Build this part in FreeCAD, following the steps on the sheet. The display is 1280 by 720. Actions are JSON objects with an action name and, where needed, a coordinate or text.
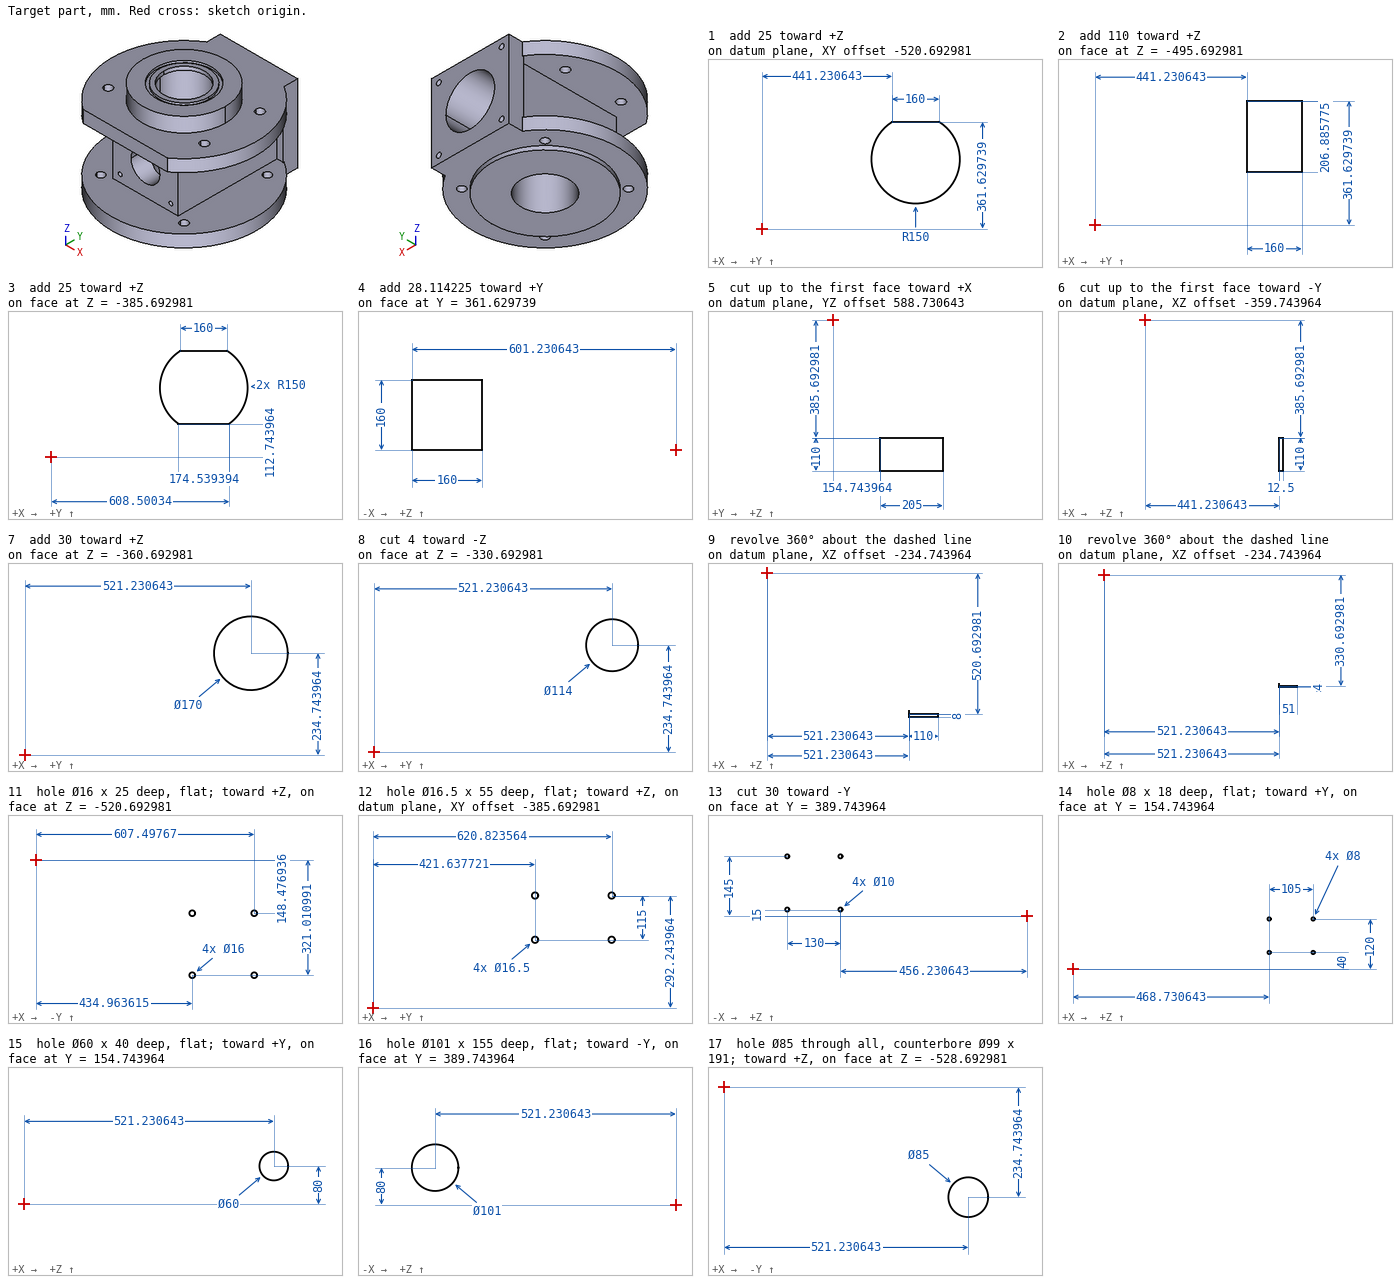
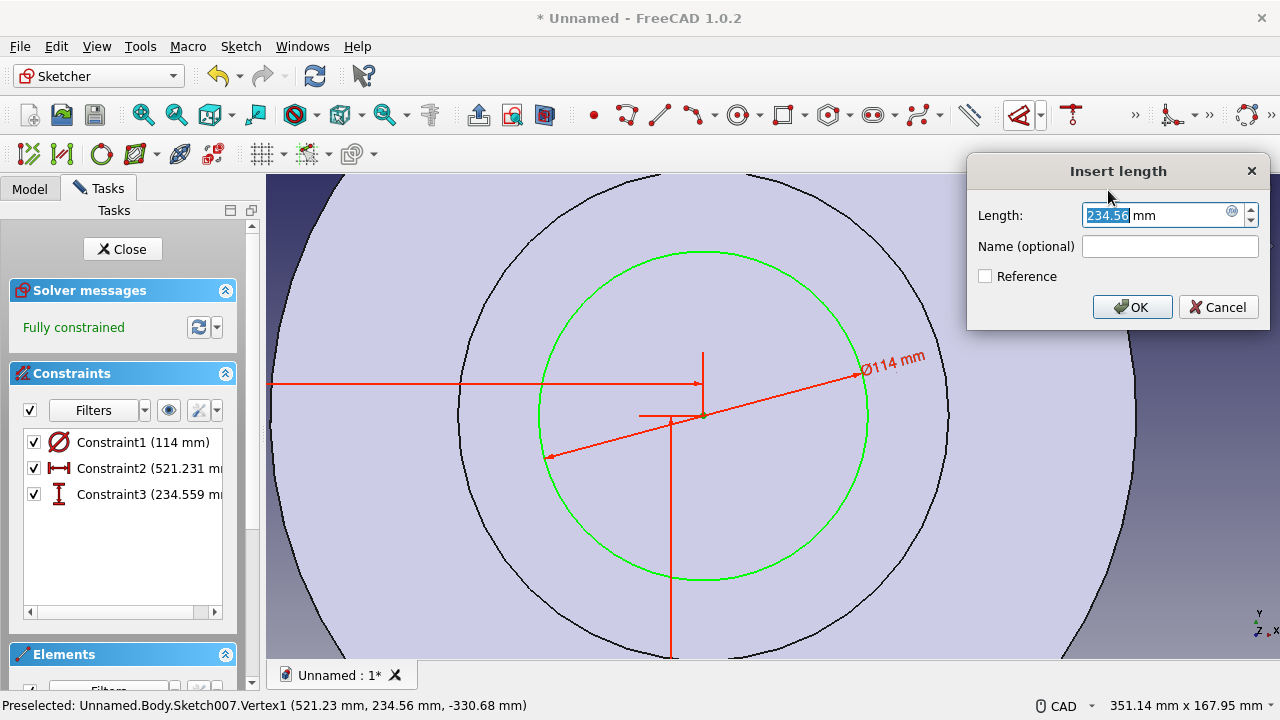
{"action": "type", "text": "234.743964"}
{"action": "key", "text": "Return"}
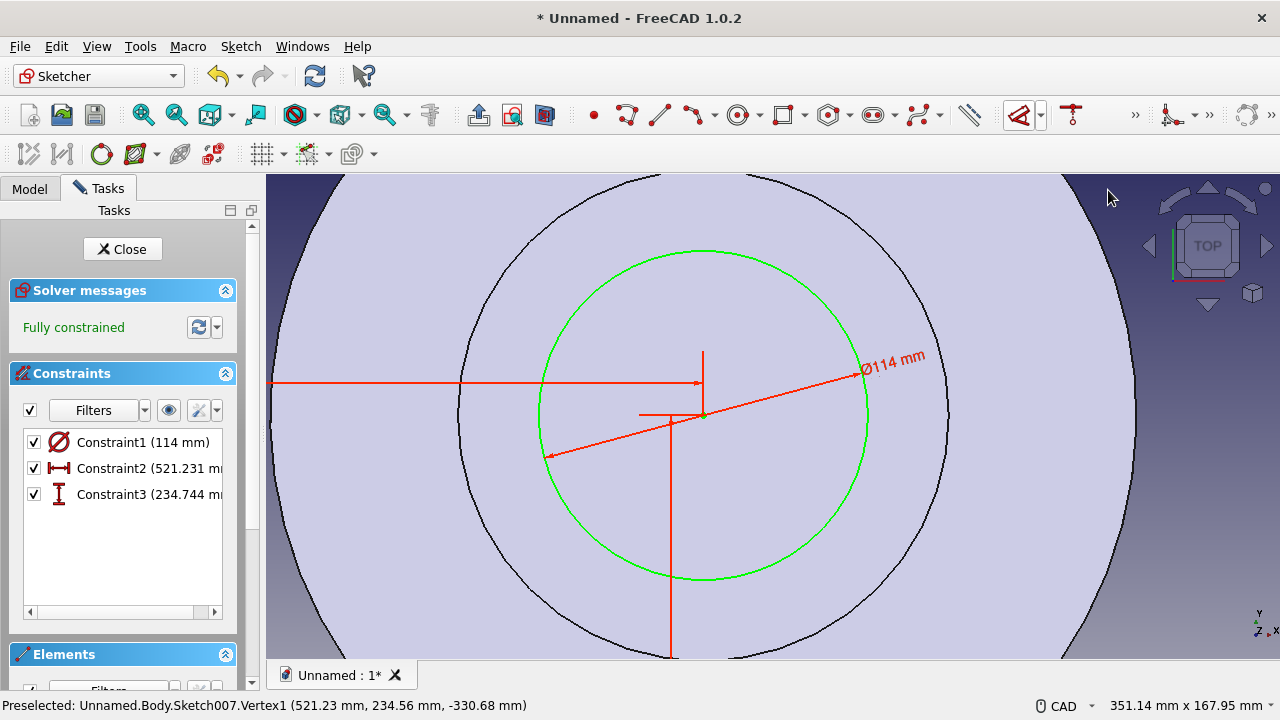
{"action": "left_click", "coordinate": [123, 249]}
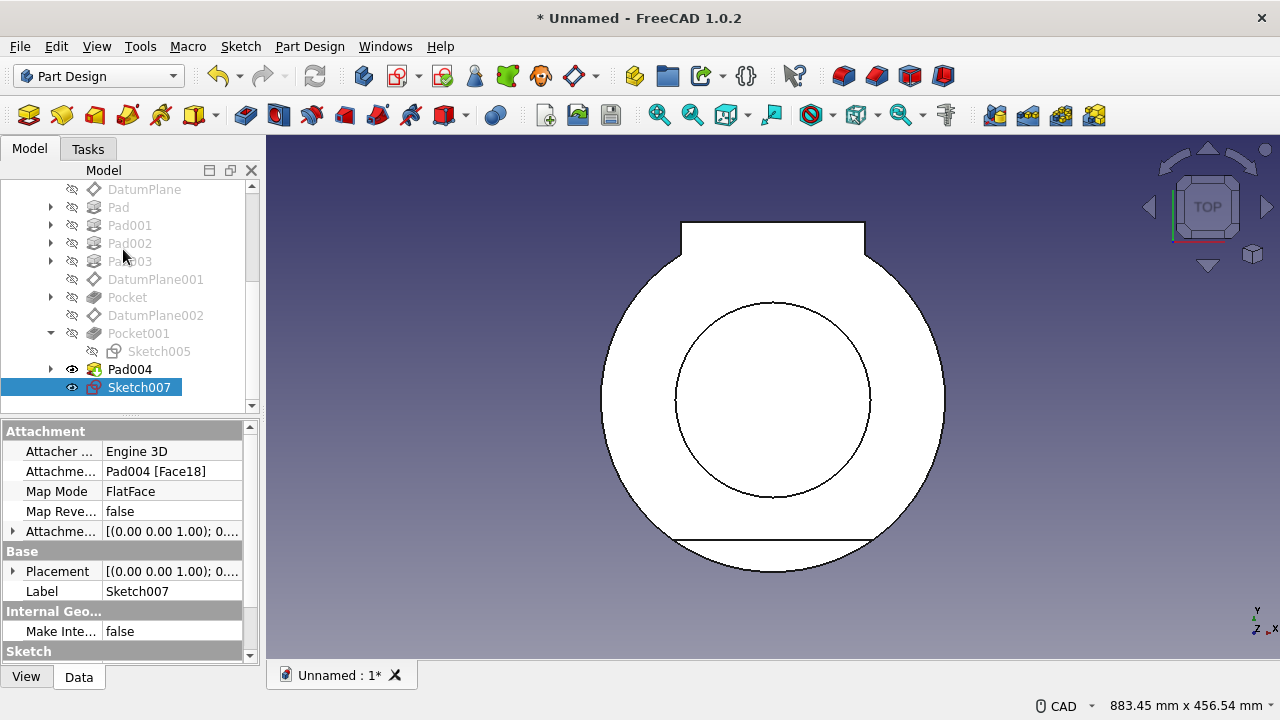
{"action": "left_click", "coordinate": [246, 116]}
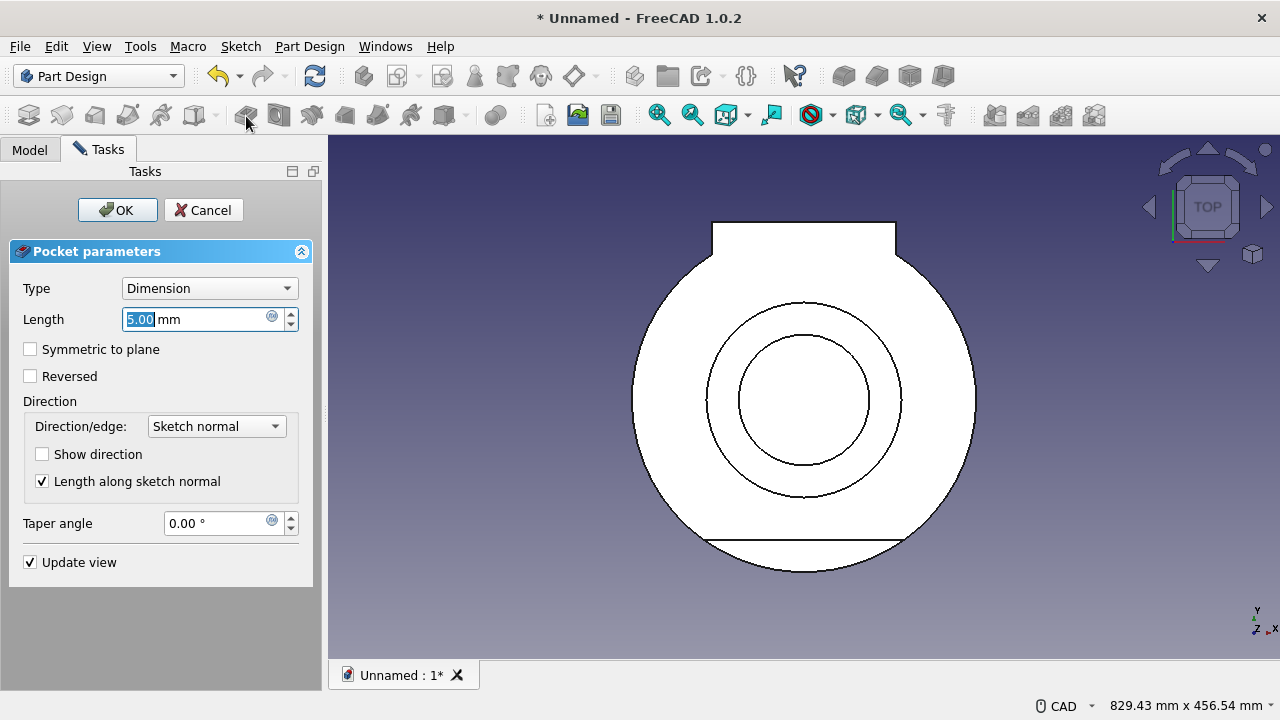
{"action": "type", "text": "4"}
{"action": "key", "text": "Tab"}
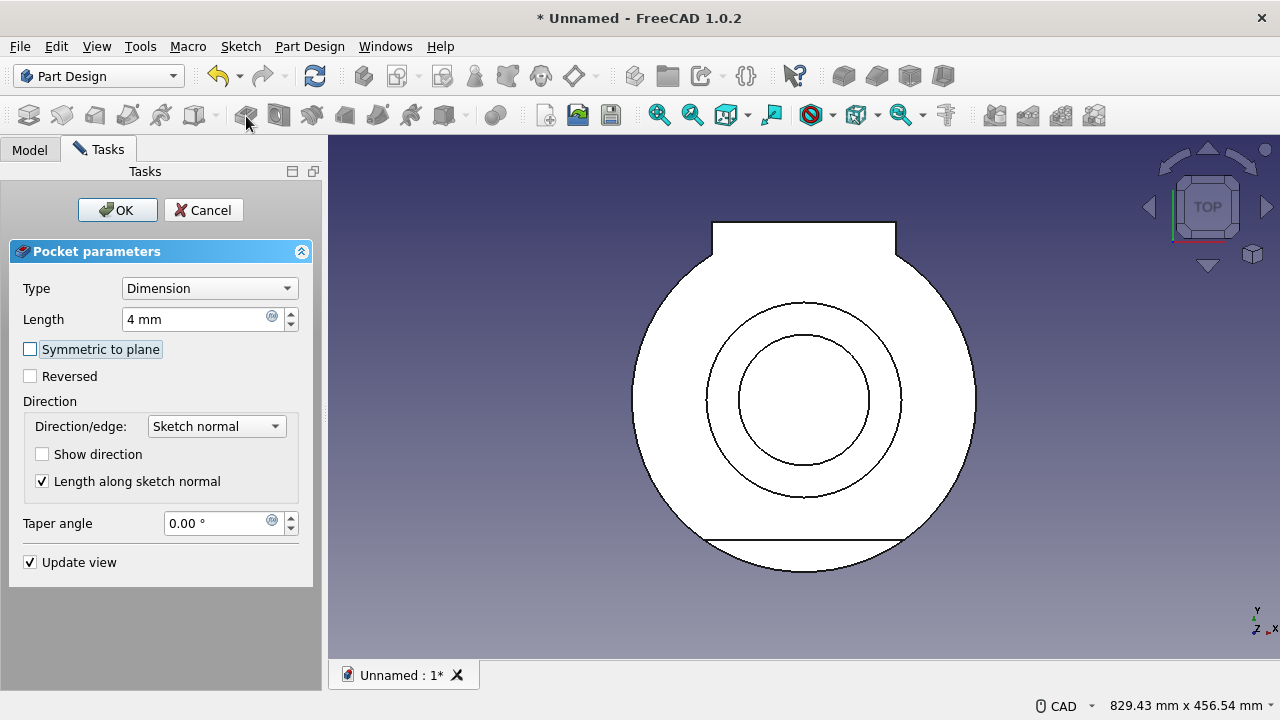
{"action": "left_click", "coordinate": [118, 210]}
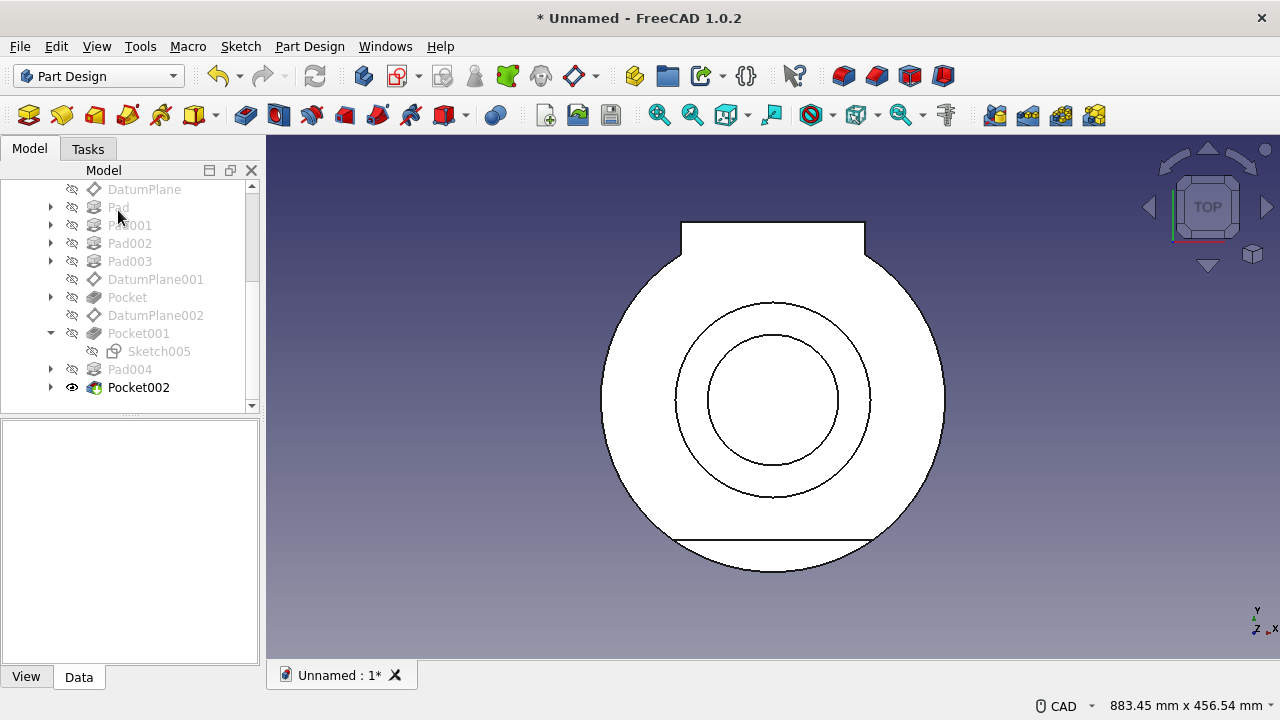
{"action": "scroll", "coordinate": [141, 293], "scroll_direction": "down", "scroll_amount": 3}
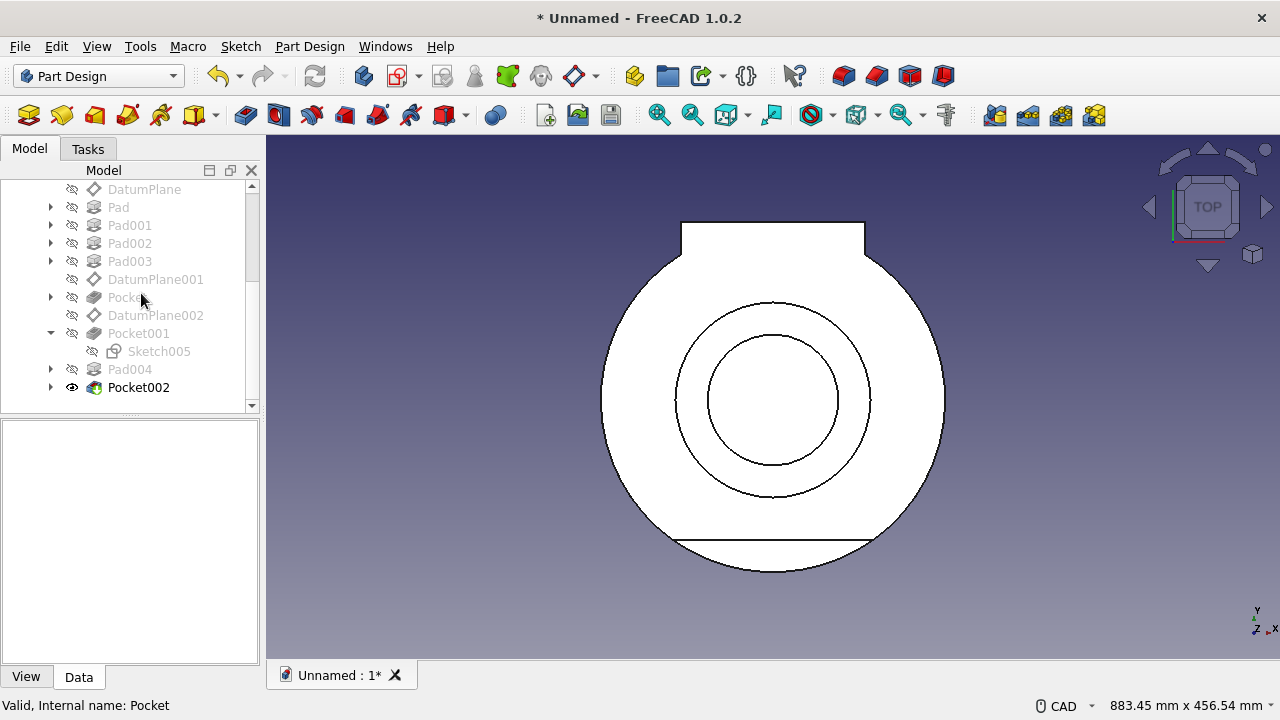
{"action": "scroll", "coordinate": [141, 293], "scroll_direction": "up", "scroll_amount": 15}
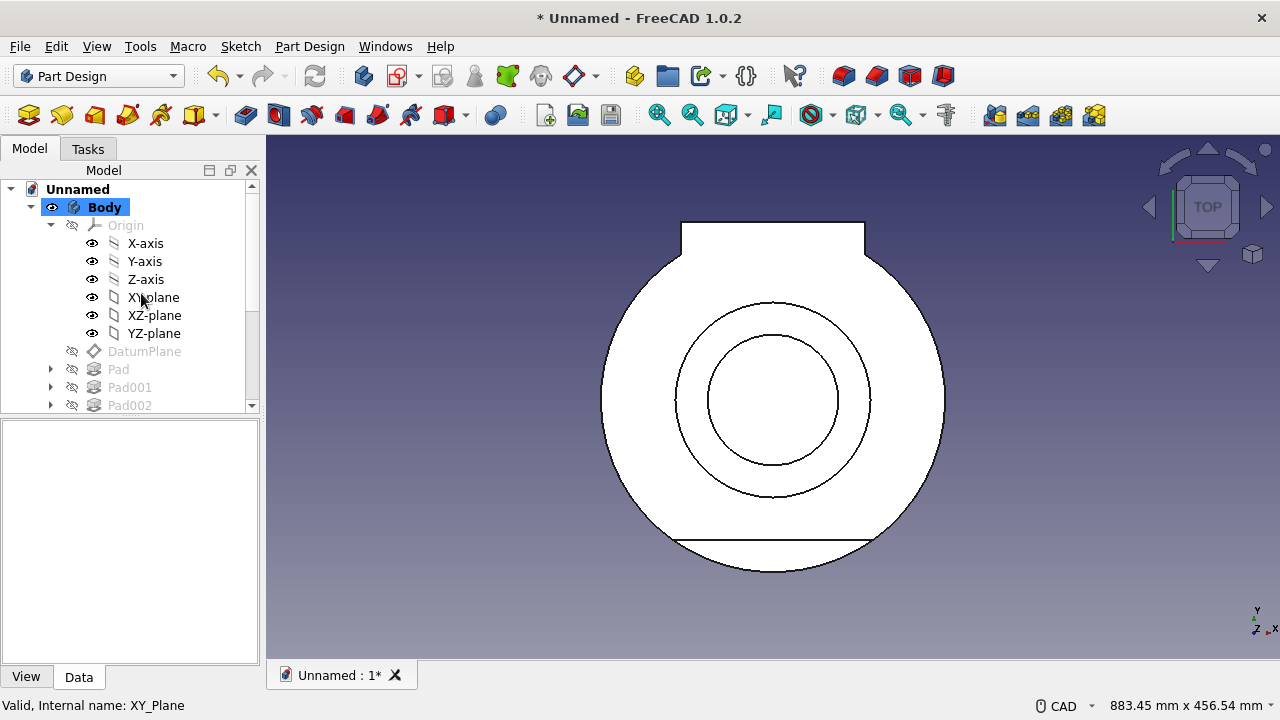
{"action": "left_click", "coordinate": [137, 315]}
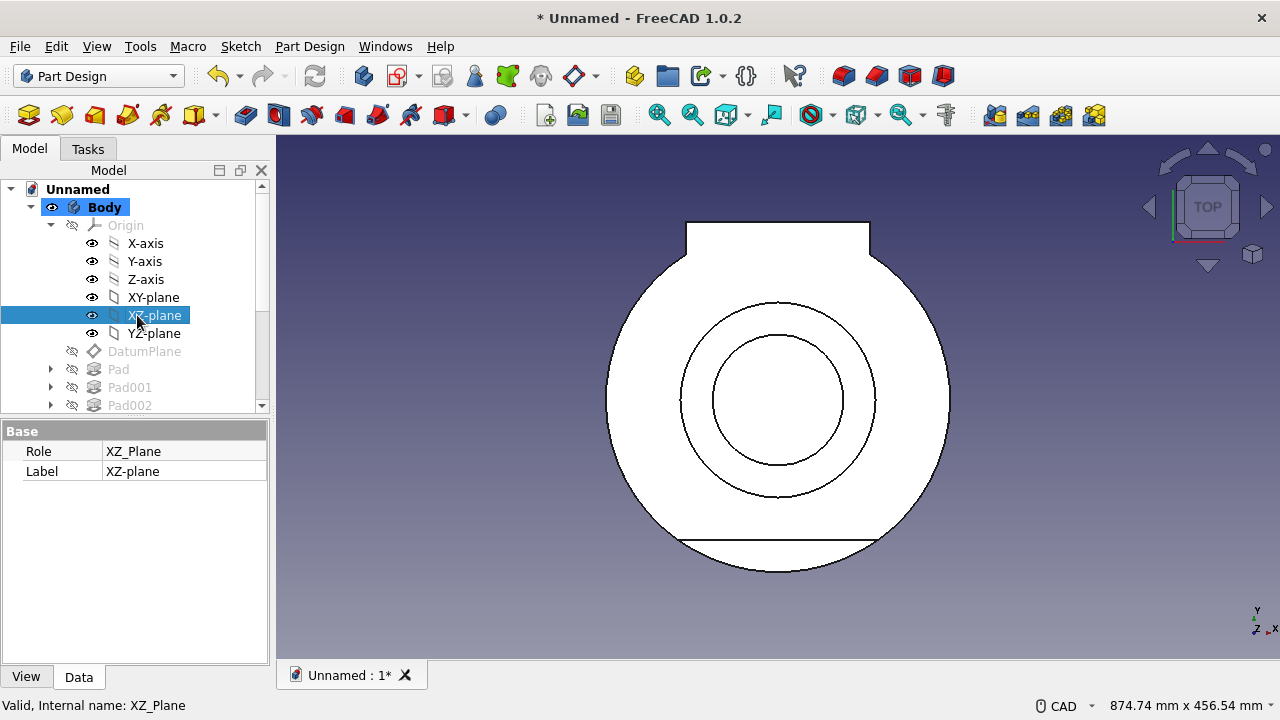
{"action": "left_click", "coordinate": [574, 76]}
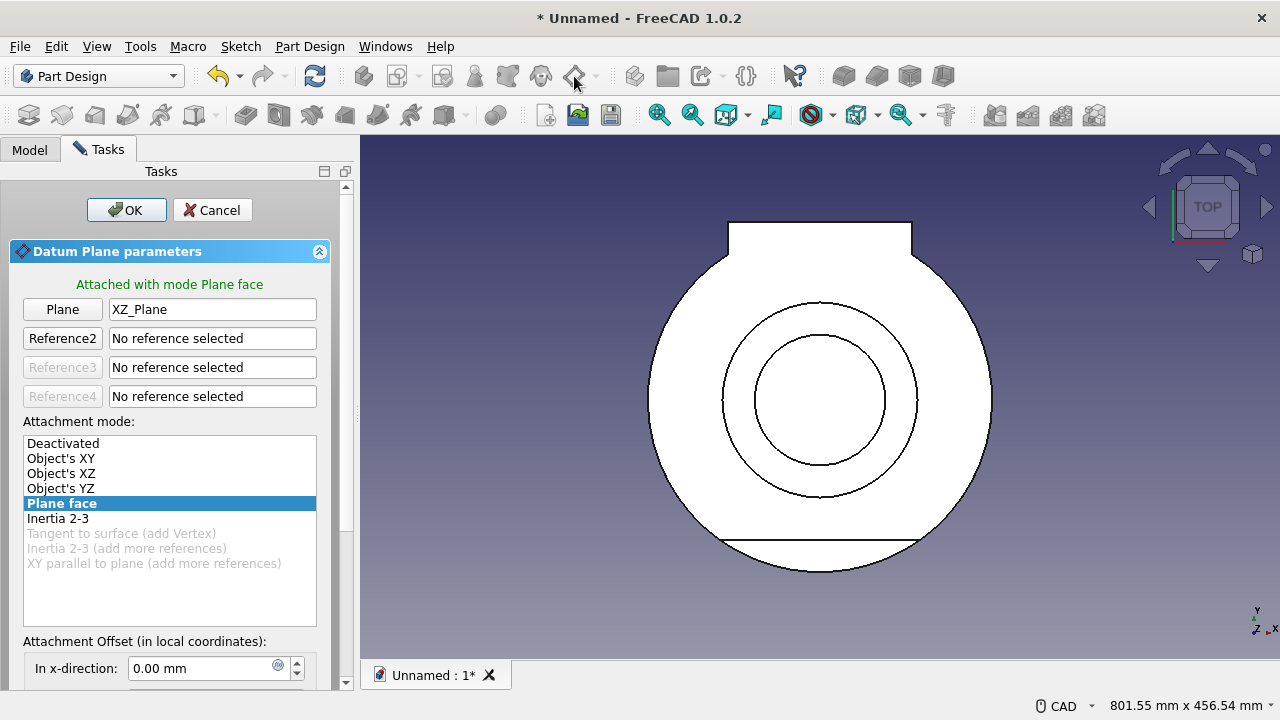
{"action": "scroll", "coordinate": [346, 436], "scroll_direction": "down", "scroll_amount": 2}